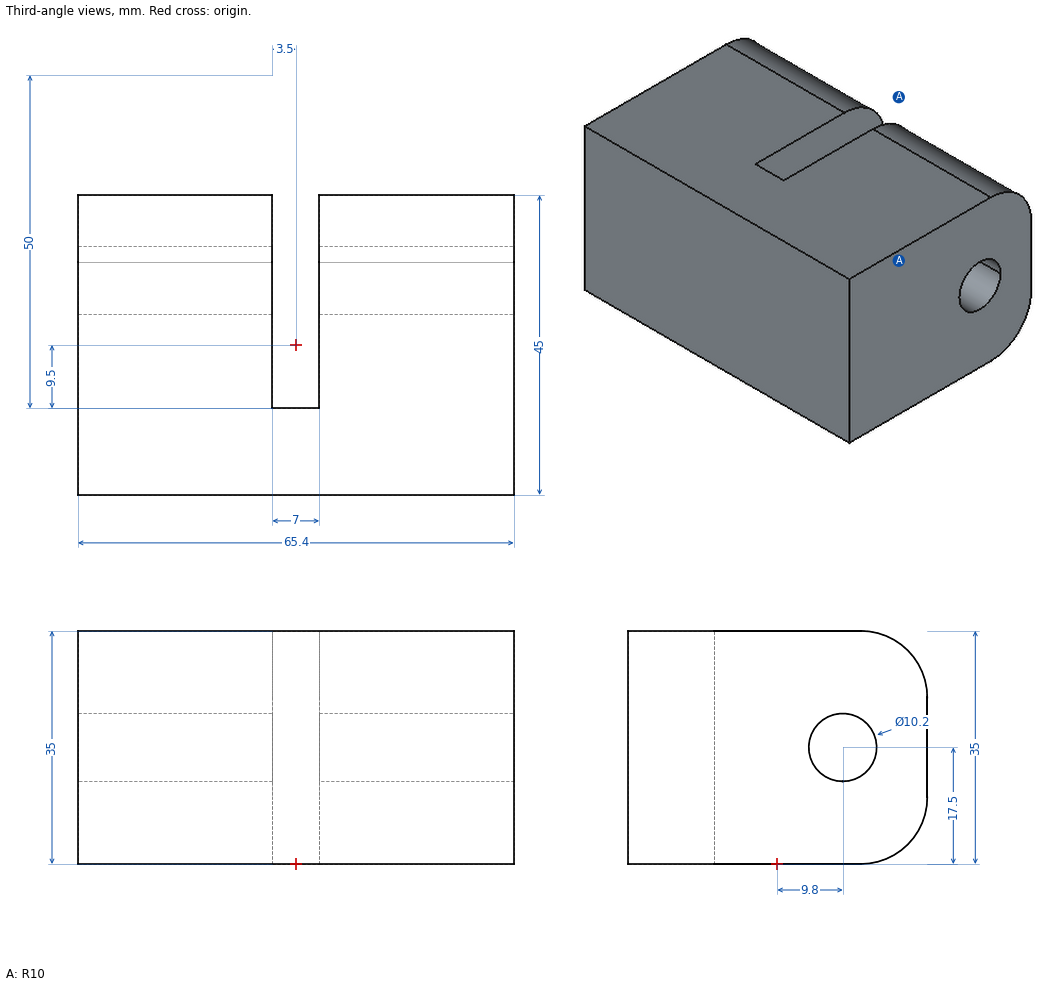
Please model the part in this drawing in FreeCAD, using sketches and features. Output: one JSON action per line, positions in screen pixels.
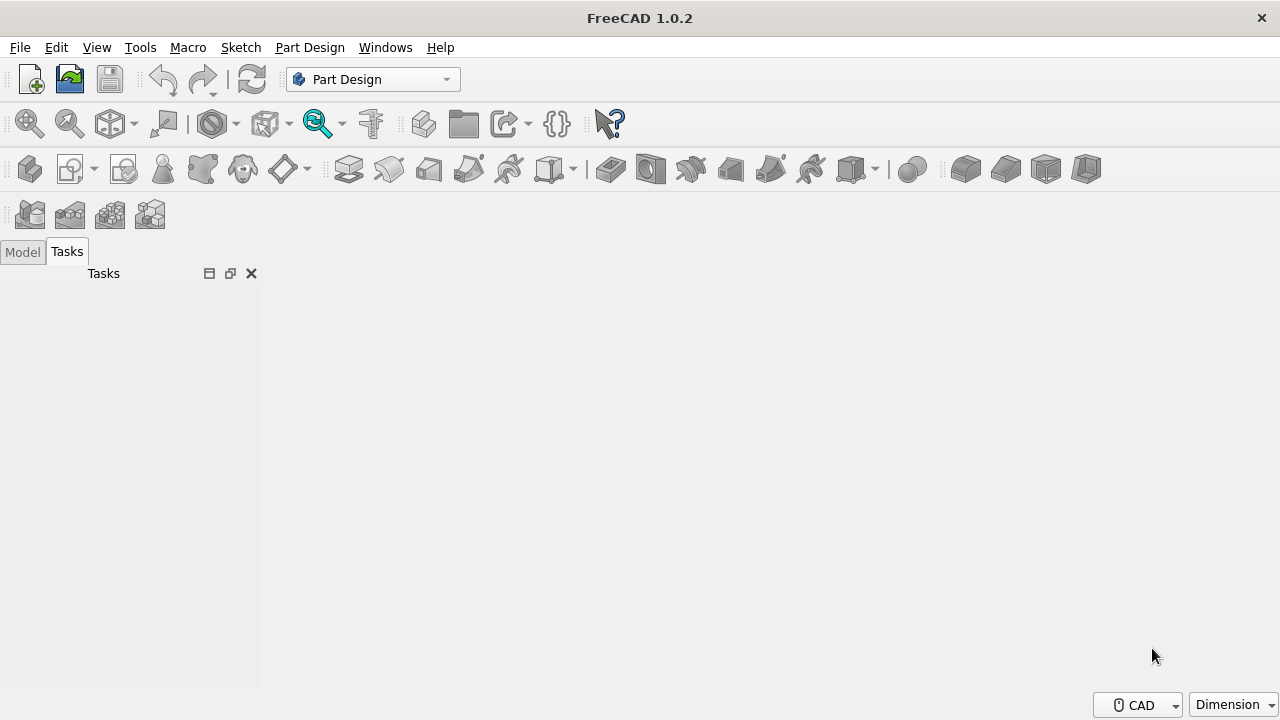
{"action": "key", "text": "ctrl+n"}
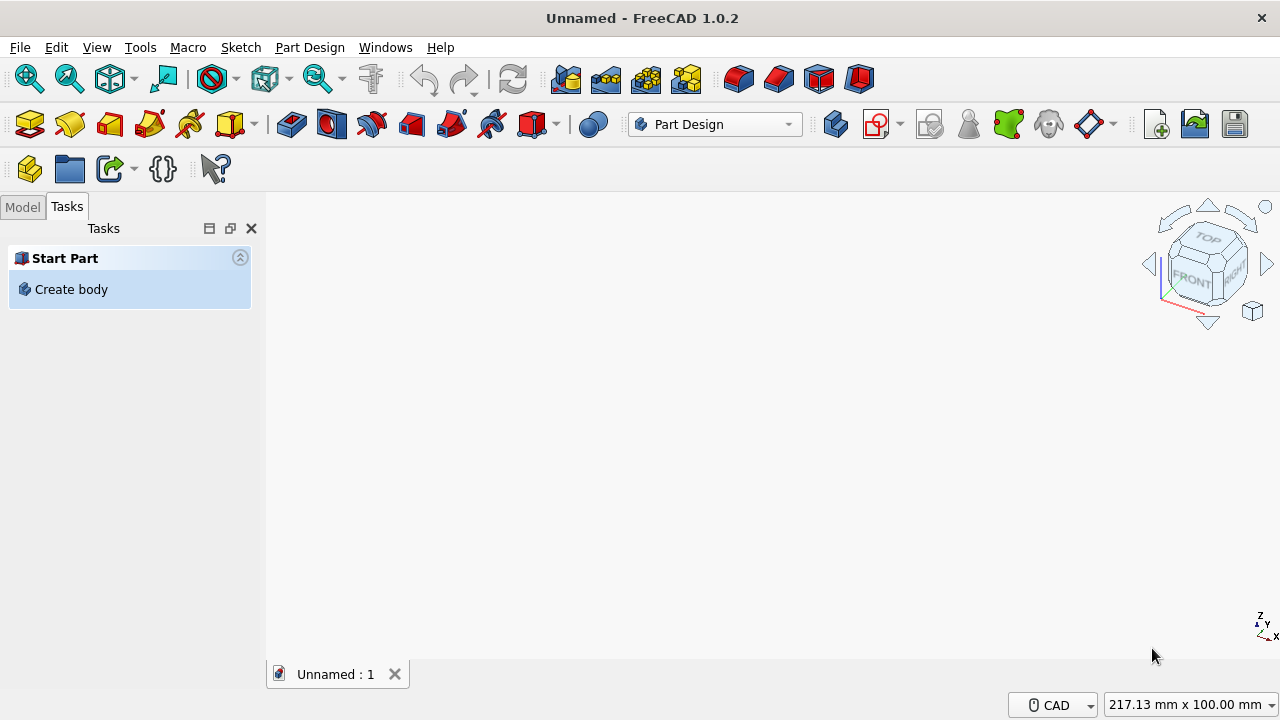
{"action": "left_click", "coordinate": [876, 124]}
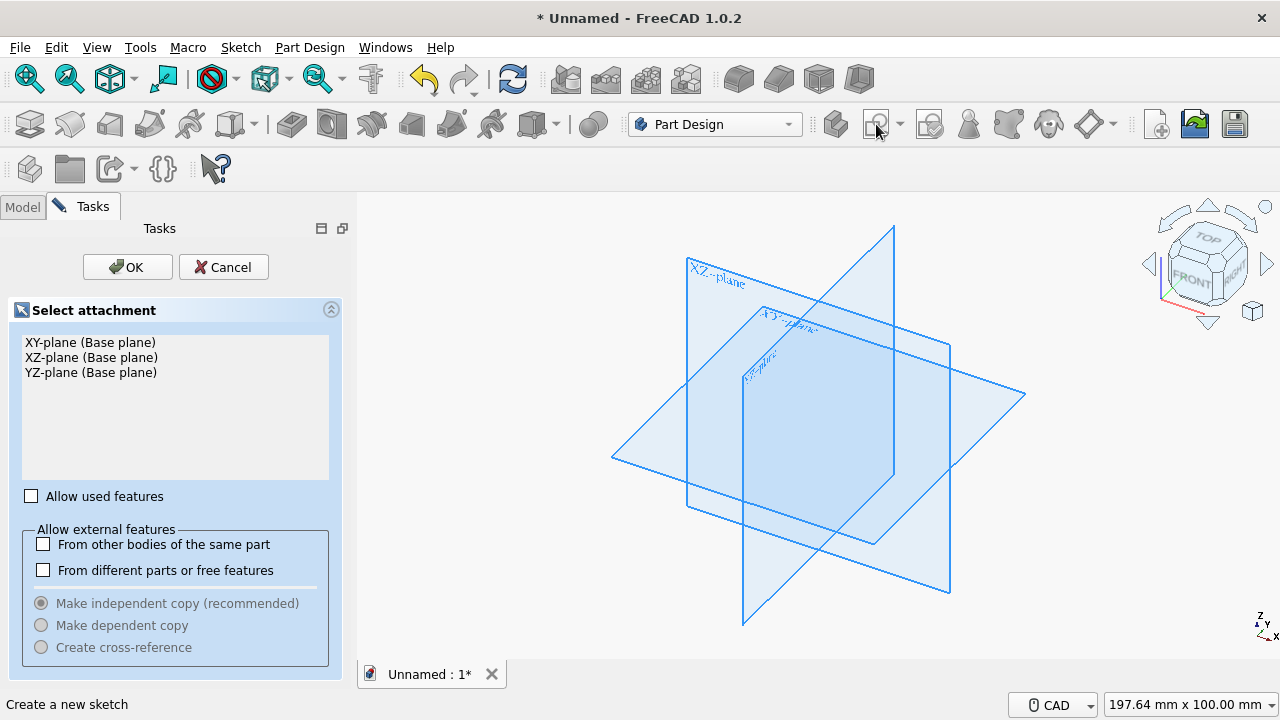
{"action": "left_click", "coordinate": [82, 342]}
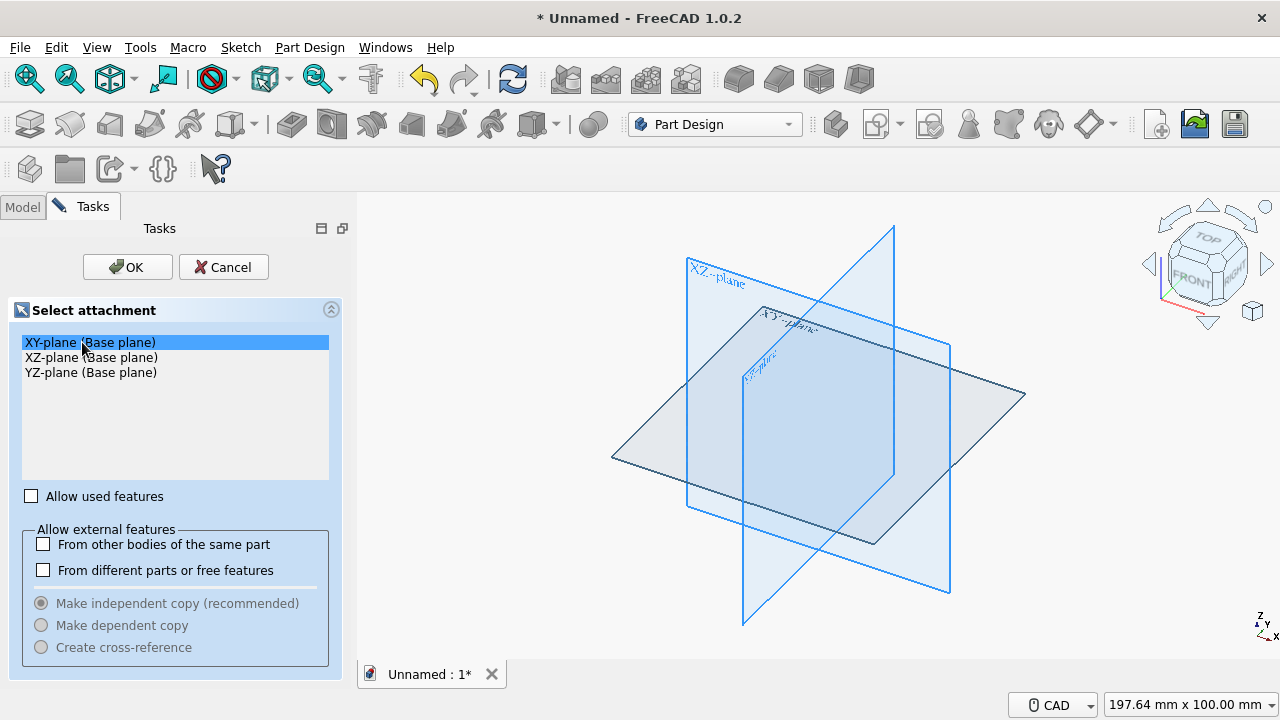
{"action": "left_click", "coordinate": [128, 267]}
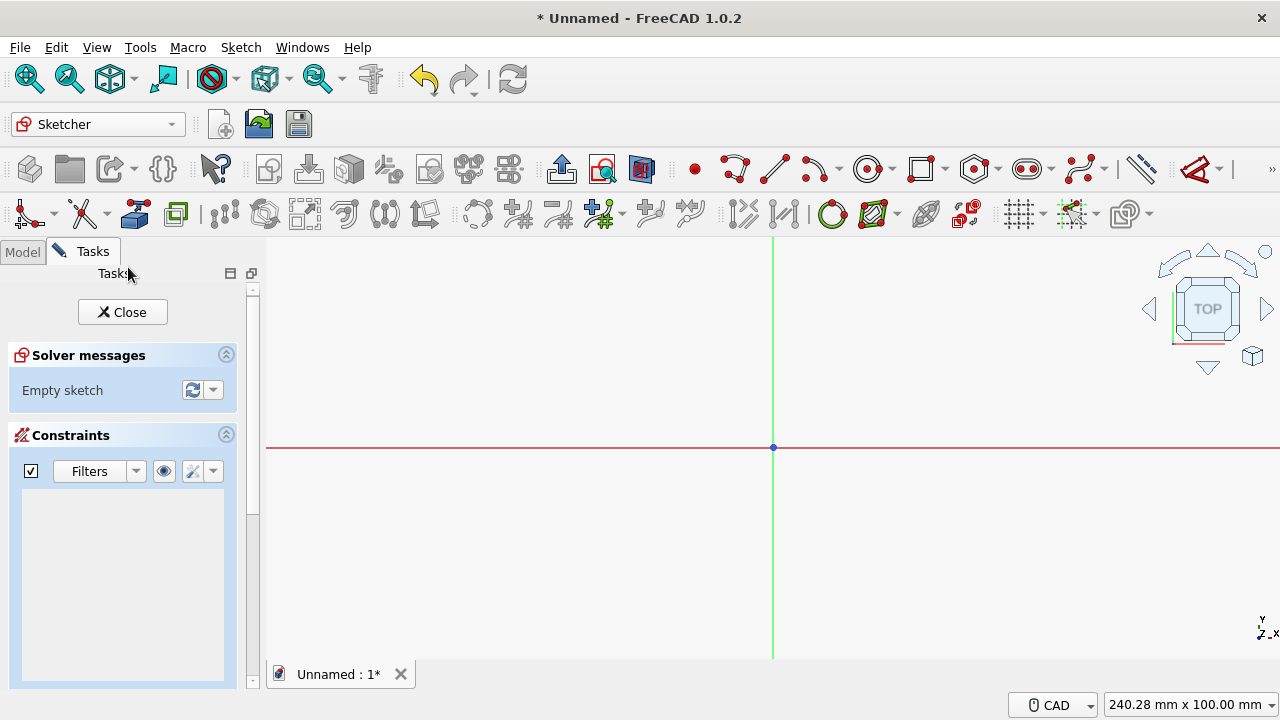
{"action": "scroll", "coordinate": [912, 448], "scroll_direction": "up", "scroll_amount": 2}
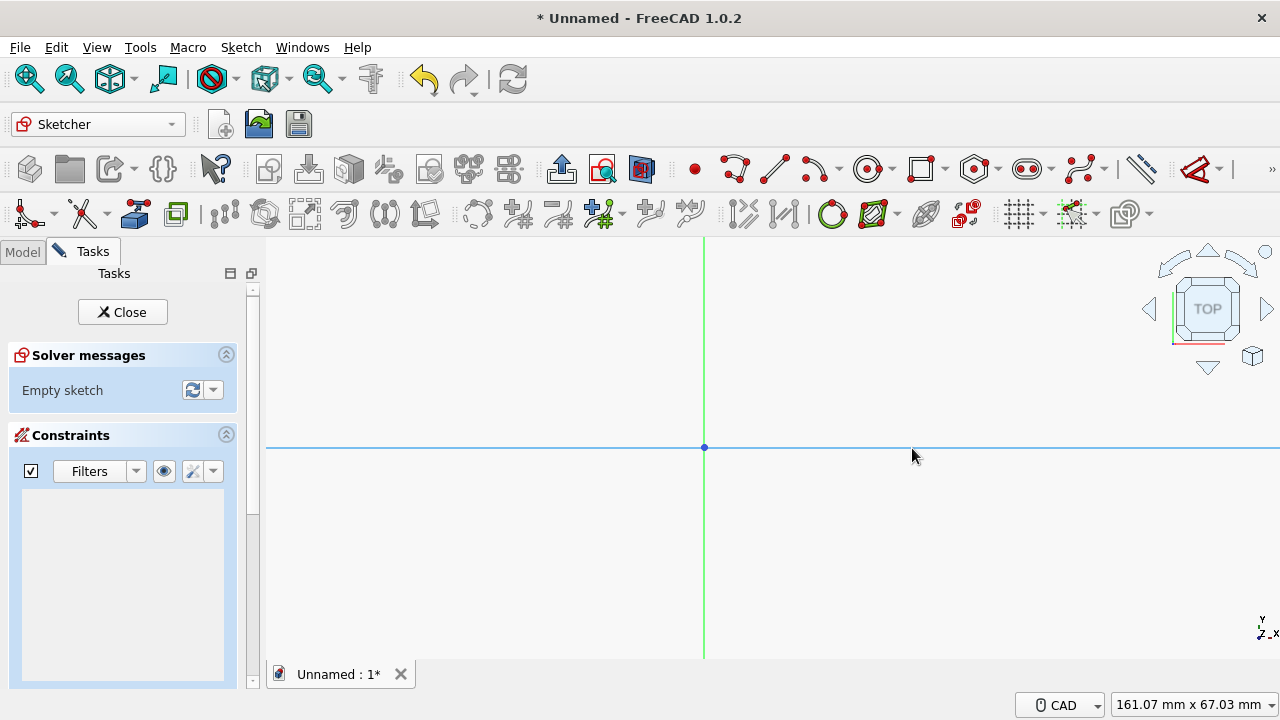
{"action": "key", "text": "g v"}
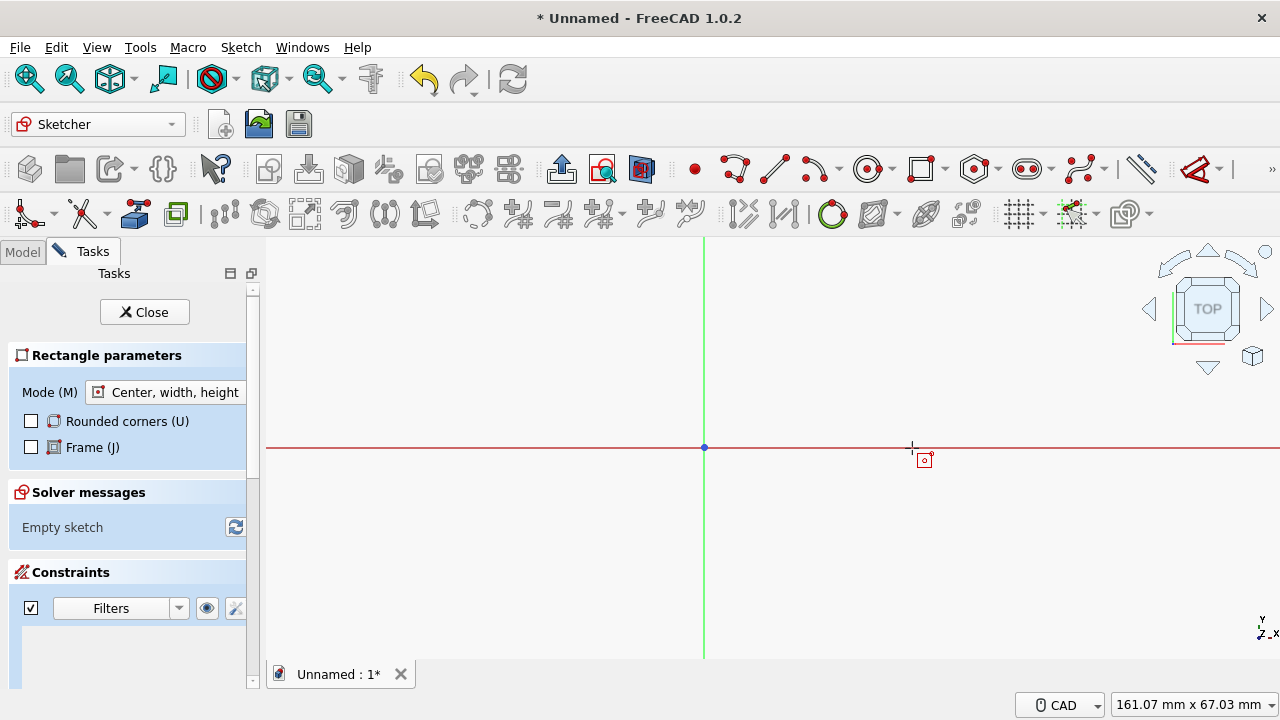
{"action": "left_click", "coordinate": [704, 448]}
{"action": "left_click", "coordinate": [910, 306]}
{"action": "key", "text": "Escape"}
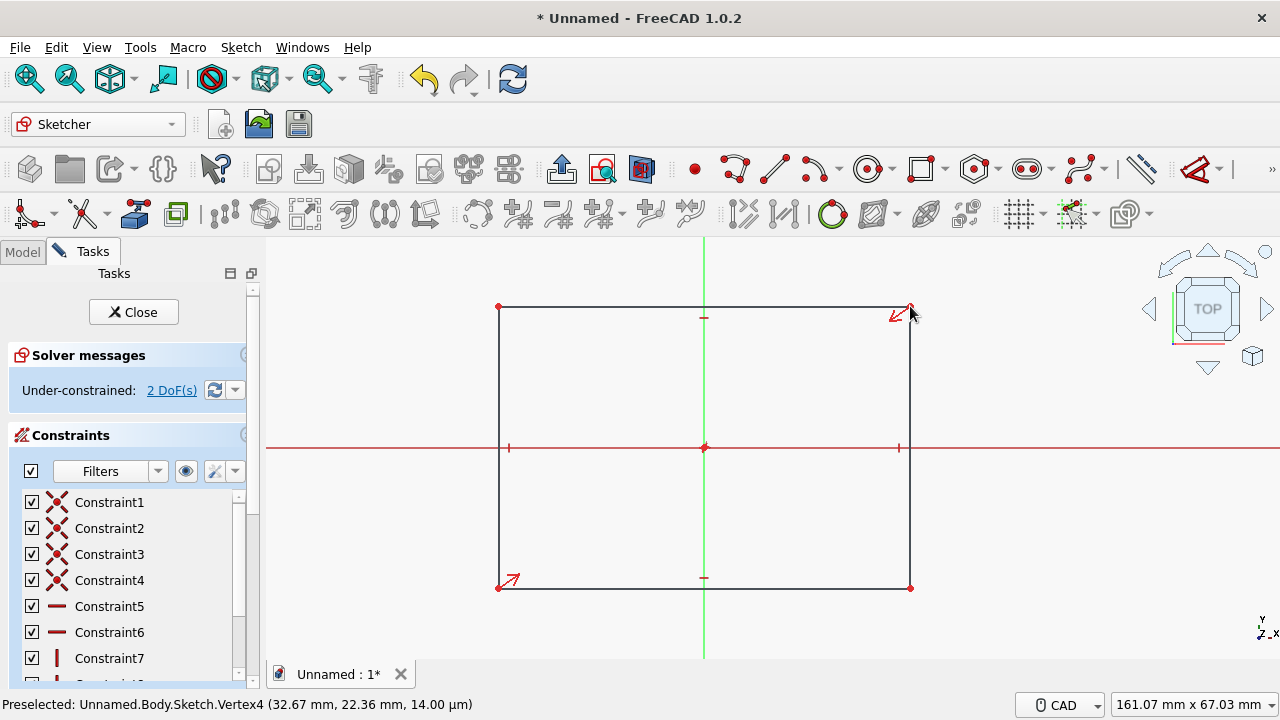
{"action": "left_click", "coordinate": [1196, 170]}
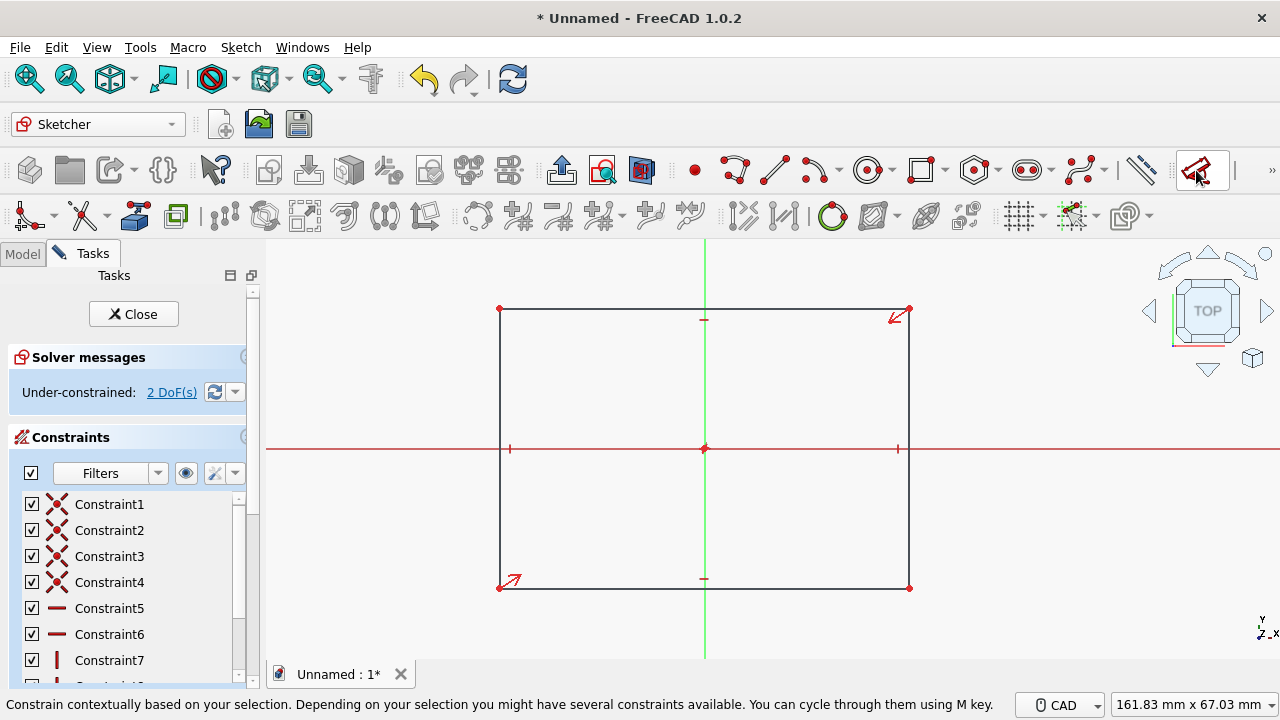
{"action": "left_click", "coordinate": [909, 505]}
{"action": "left_click", "coordinate": [943, 384]}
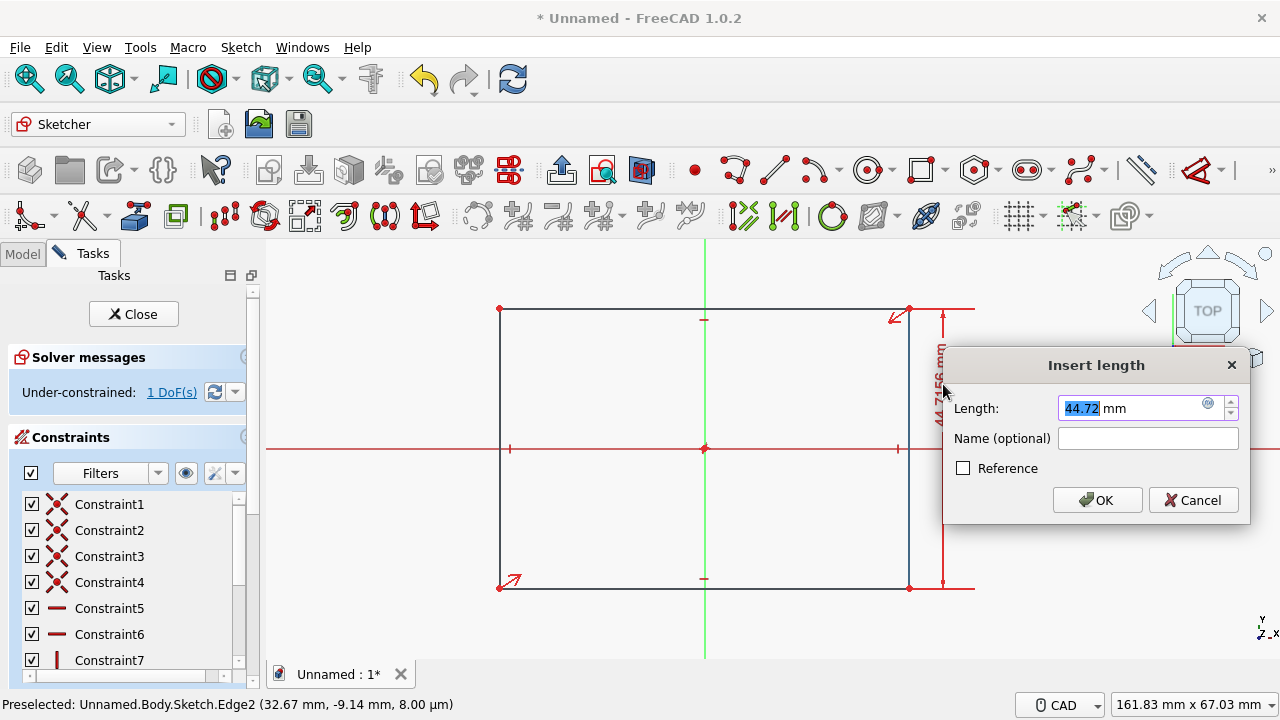
{"action": "type", "text": "45"}
{"action": "key", "text": "Return"}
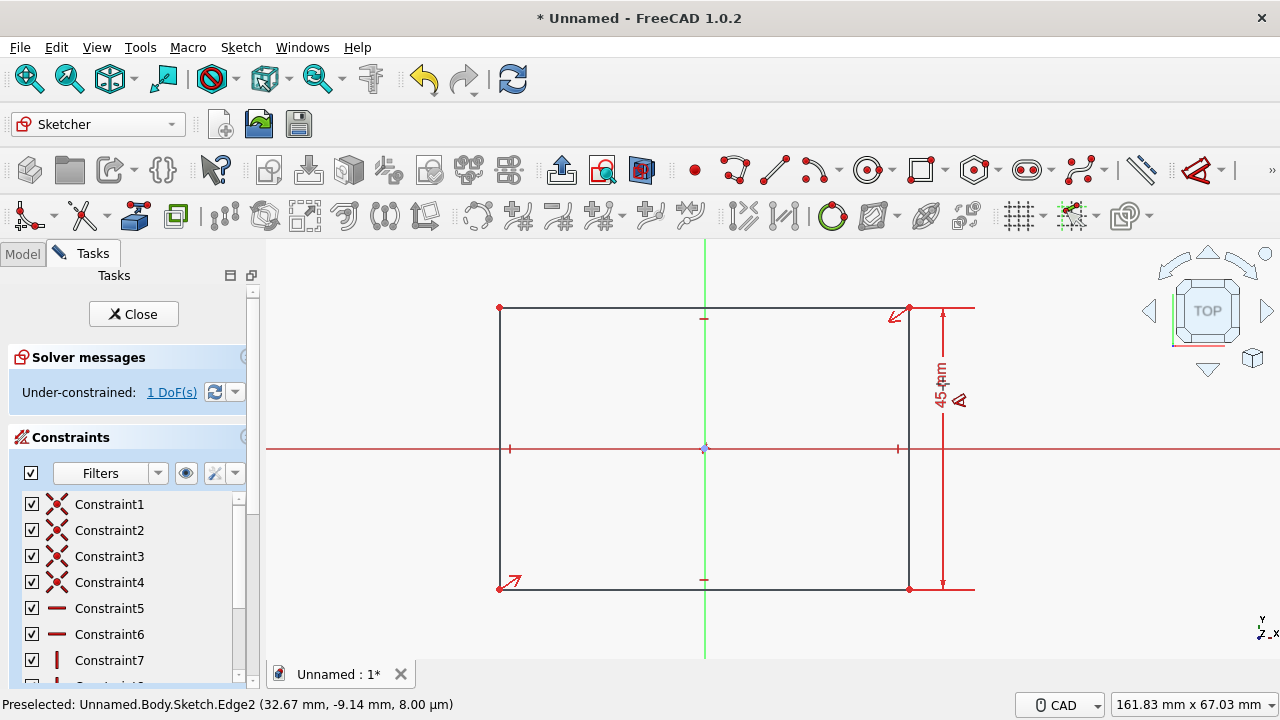
{"action": "left_click", "coordinate": [623, 590]}
{"action": "left_click", "coordinate": [610, 624]}